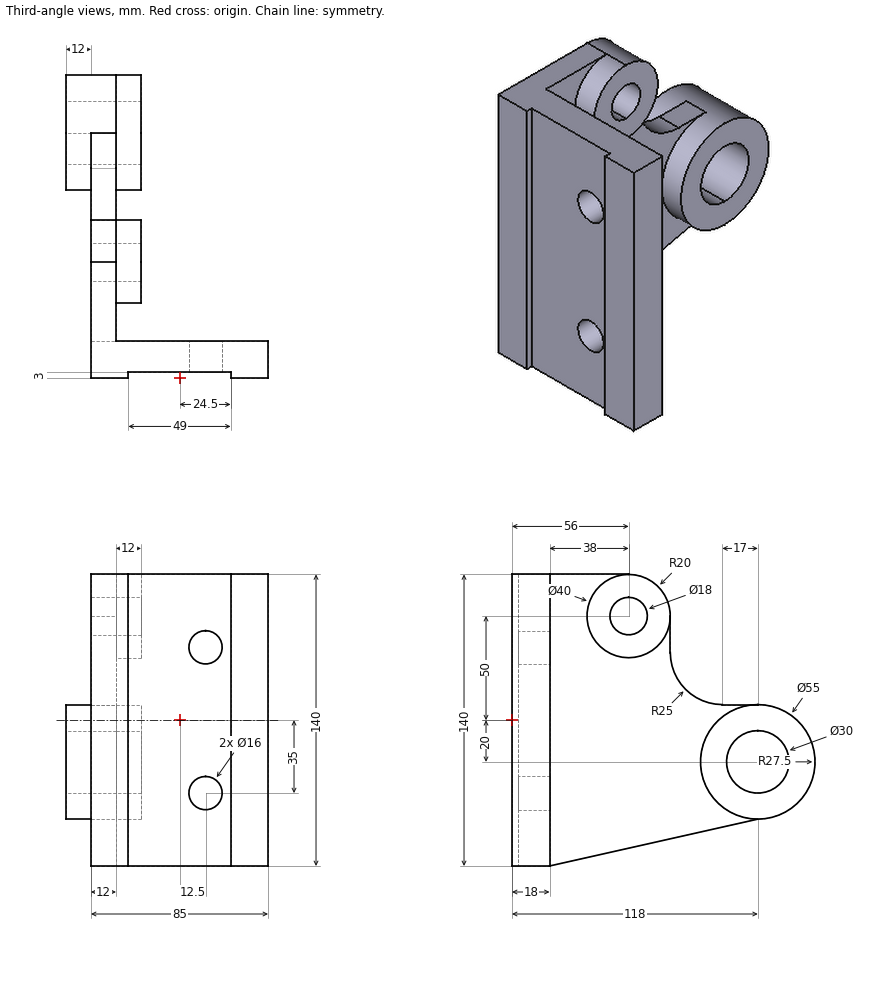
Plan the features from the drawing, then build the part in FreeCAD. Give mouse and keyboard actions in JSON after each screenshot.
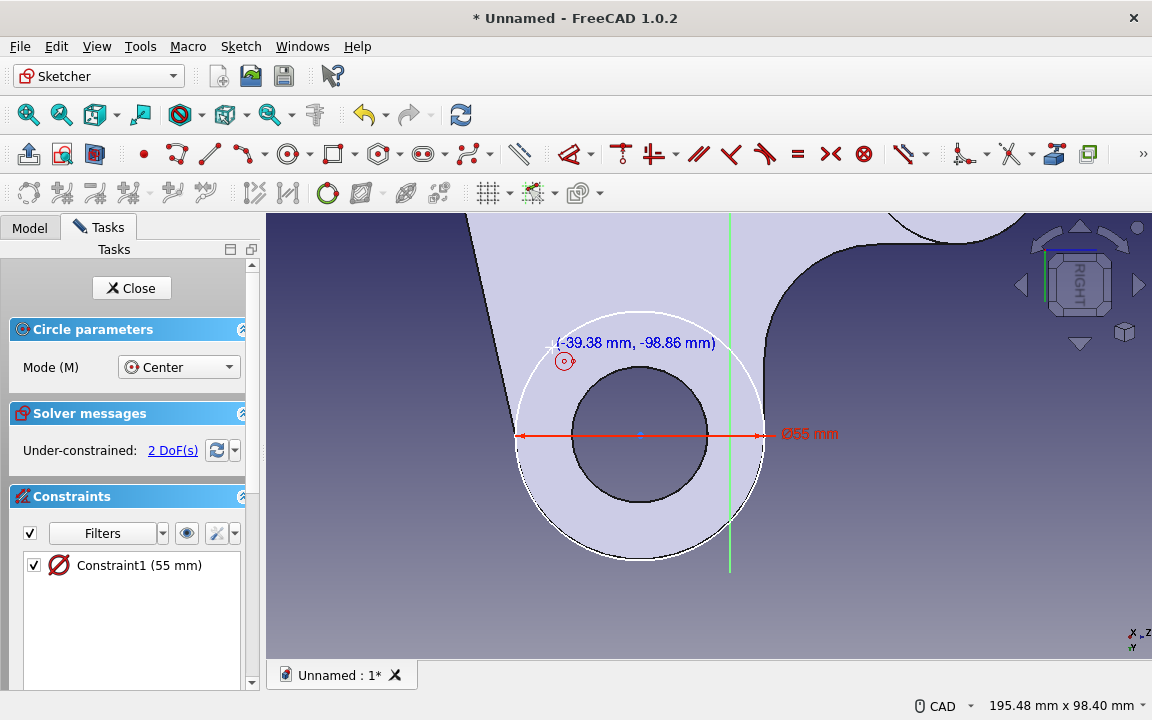
{"action": "left_click", "coordinate": [640, 436]}
{"action": "mouse_move", "coordinate": [688, 387]}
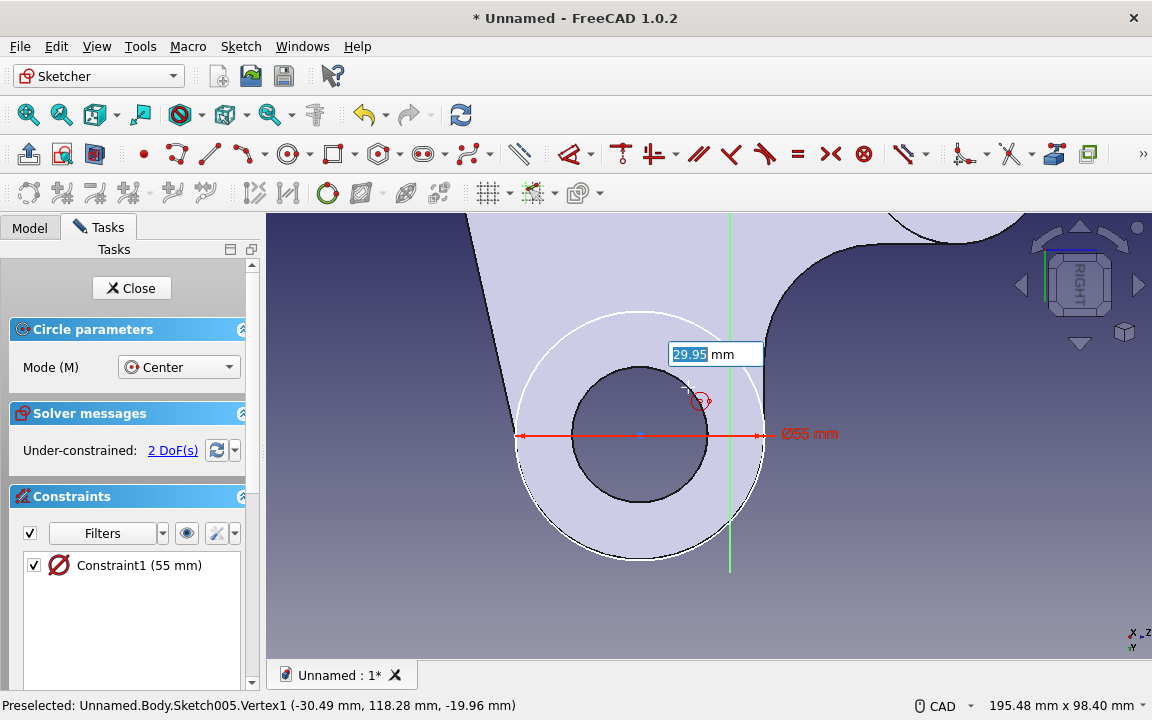
{"action": "type", "text": "30"}
{"action": "key", "text": "Return"}
{"action": "key", "text": "Escape"}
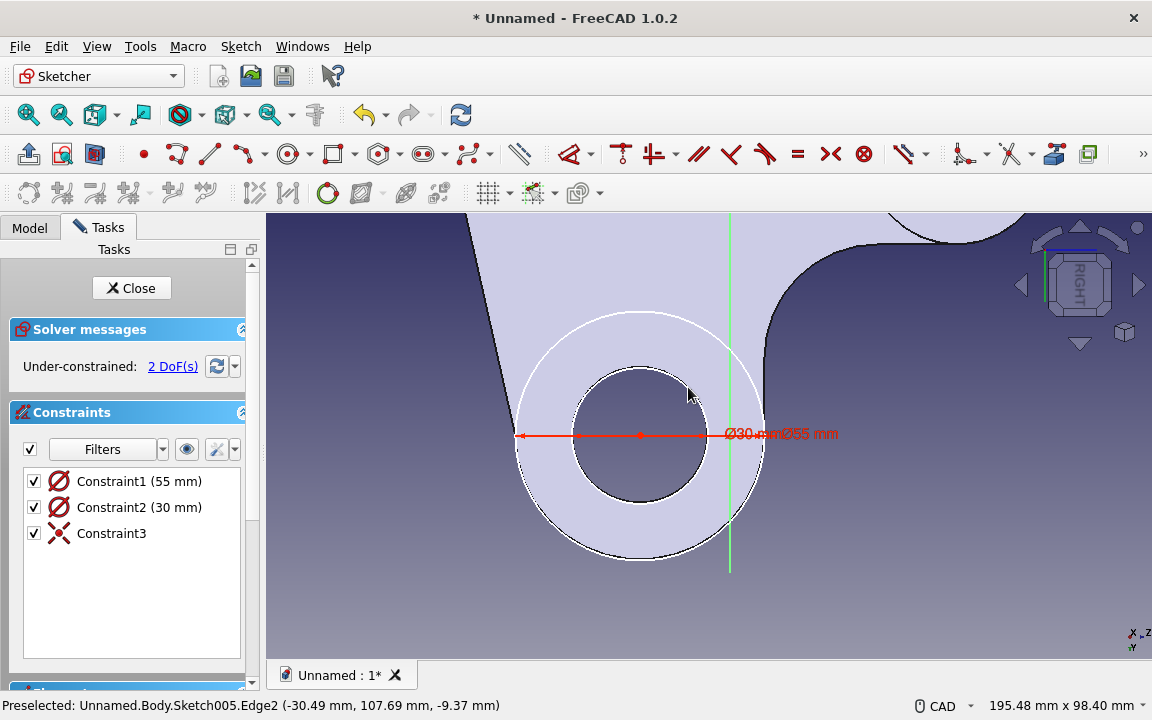
{"action": "left_click", "coordinate": [568, 154]}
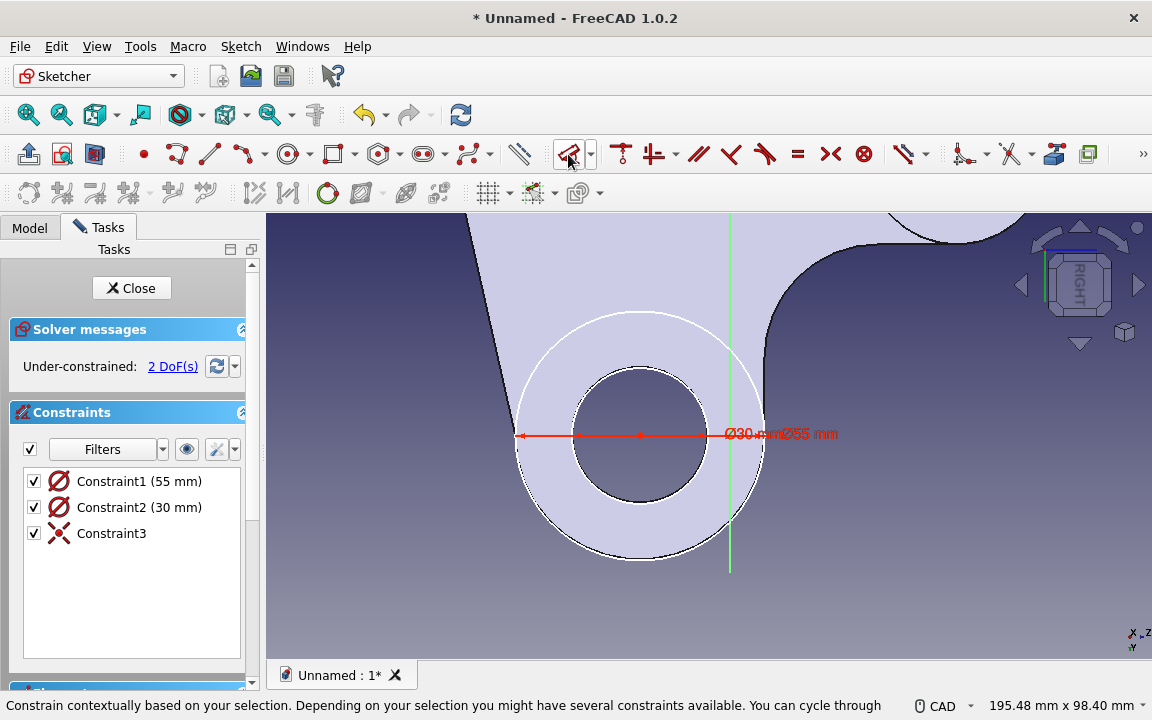
{"action": "left_click", "coordinate": [640, 436]}
{"action": "left_click", "coordinate": [664, 470]}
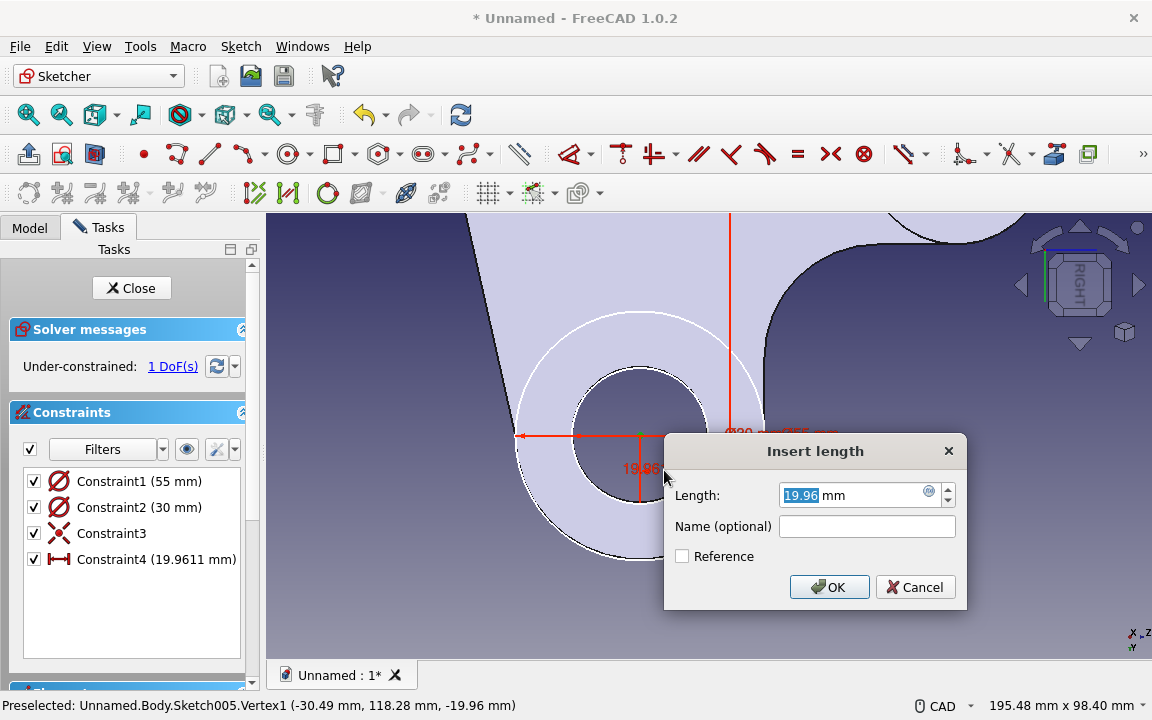
{"action": "type", "text": "20"}
{"action": "key", "text": "Return"}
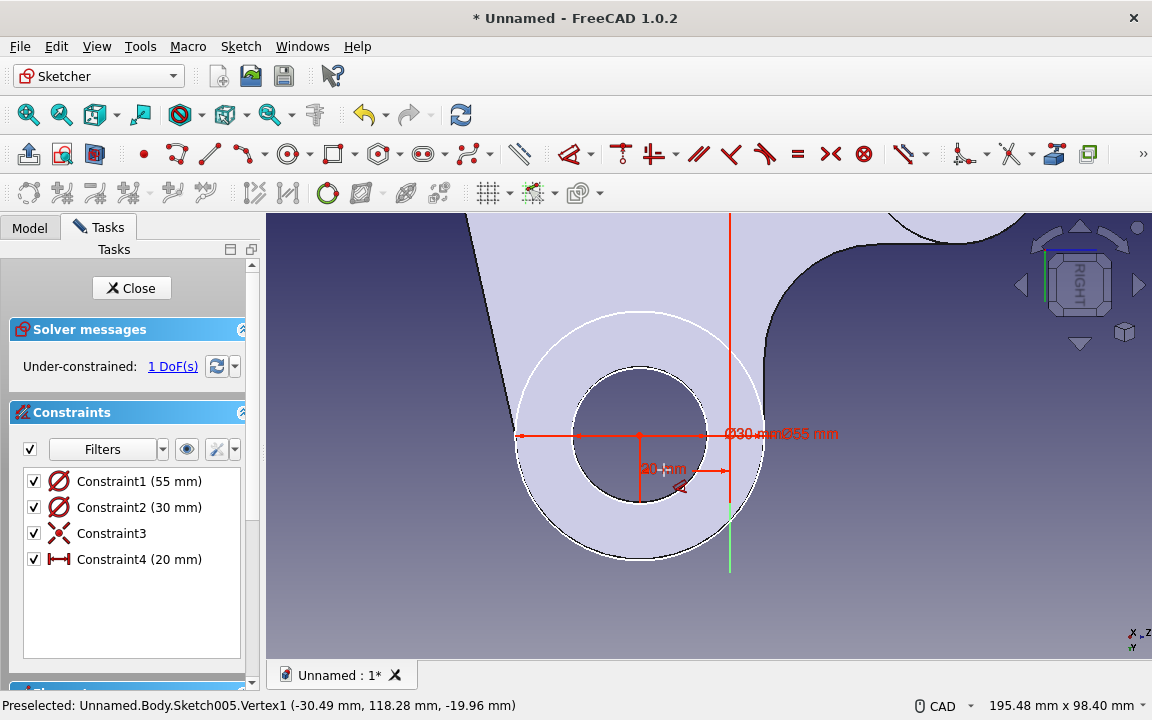
{"action": "left_click", "coordinate": [640, 436]}
{"action": "left_click", "coordinate": [764, 339]}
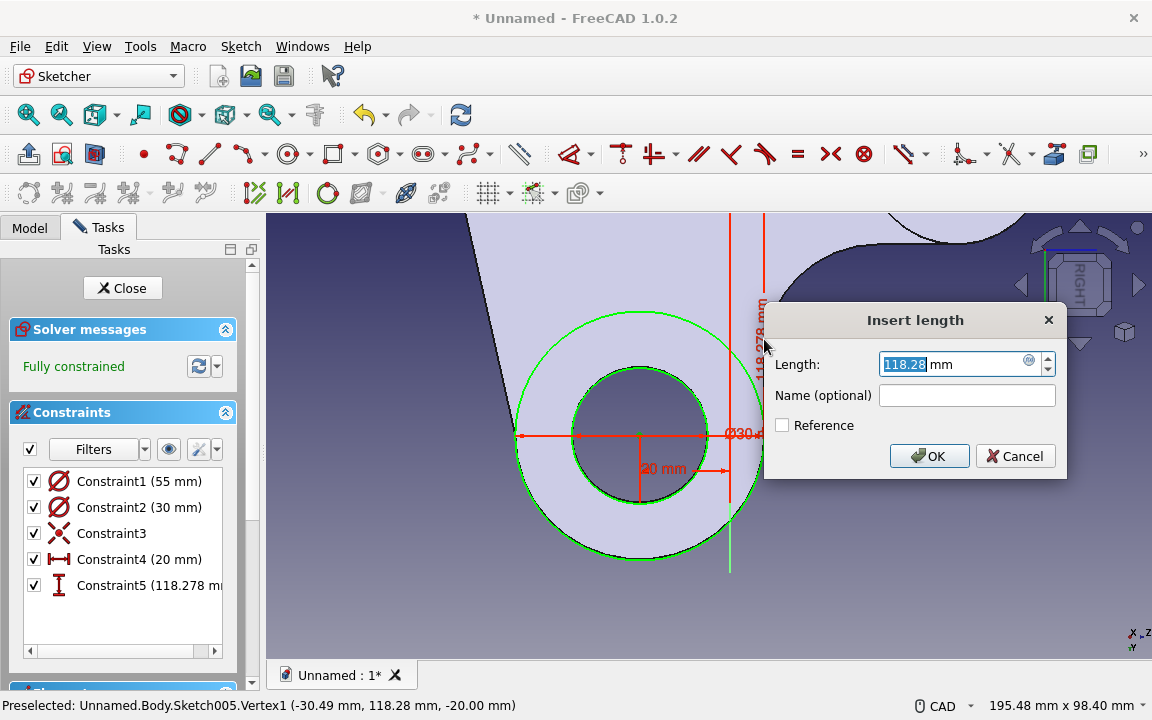
{"action": "type", "text": "118"}
{"action": "key", "text": "Return"}
{"action": "key", "text": "Escape"}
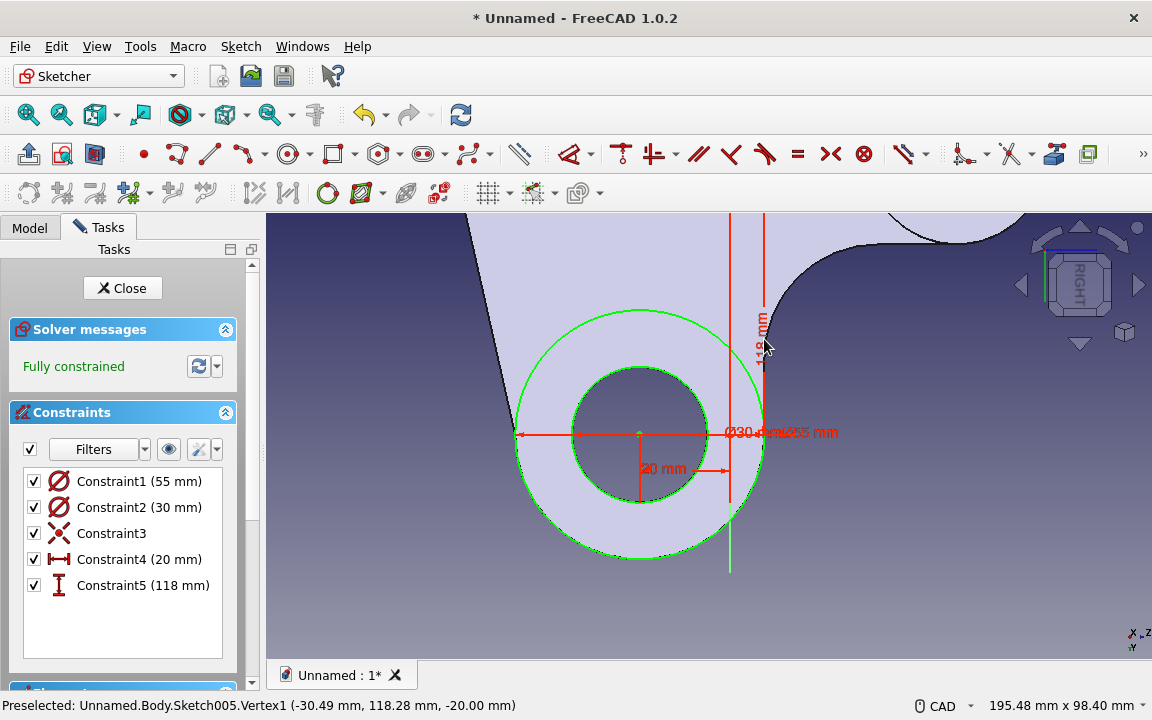
{"action": "left_click", "coordinate": [123, 288]}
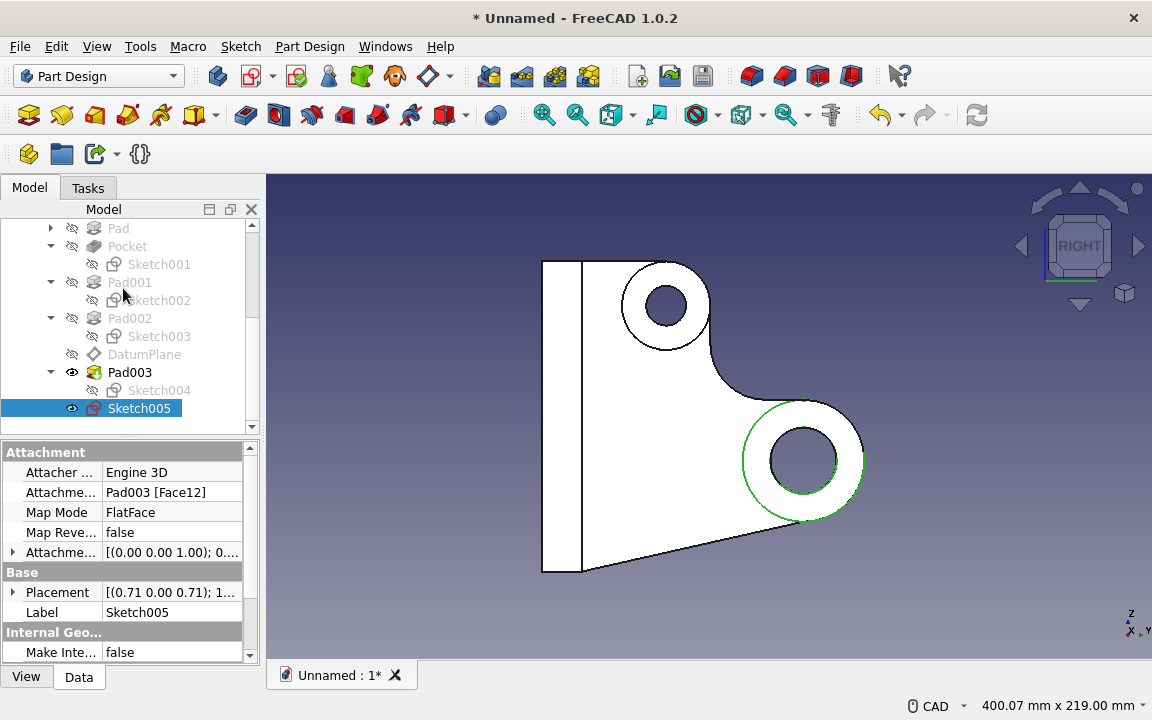
{"action": "left_click", "coordinate": [29, 116]}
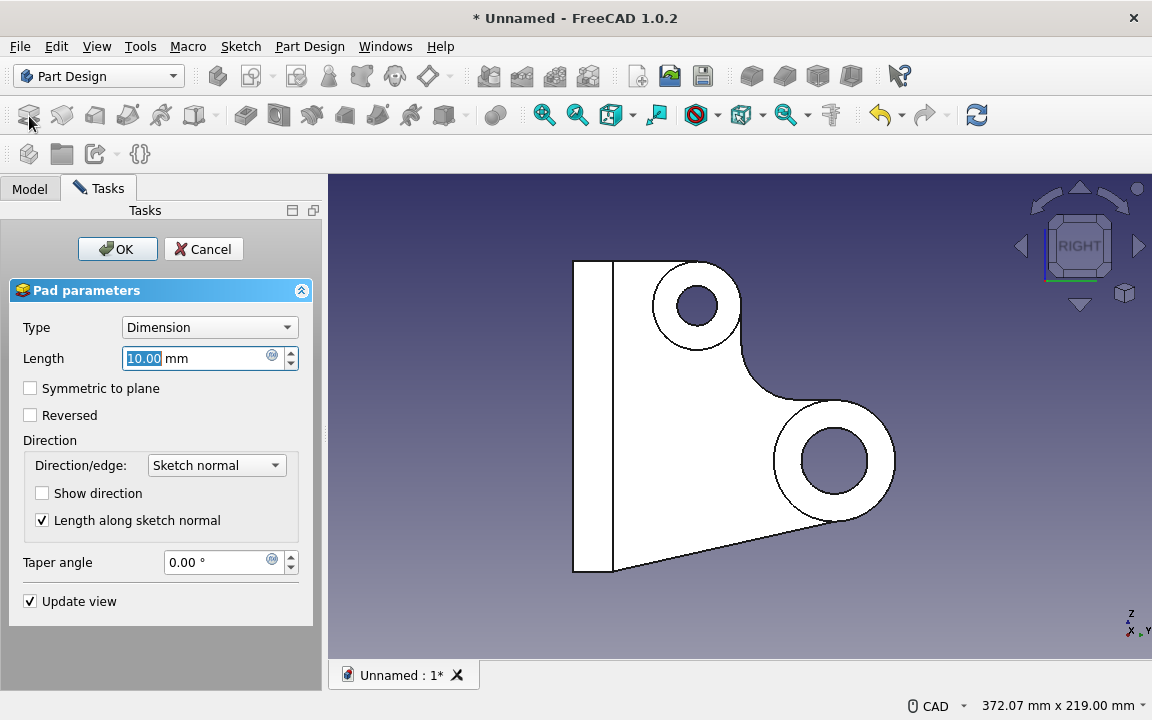
{"action": "type", "text": "12"}
{"action": "key", "text": "Tab"}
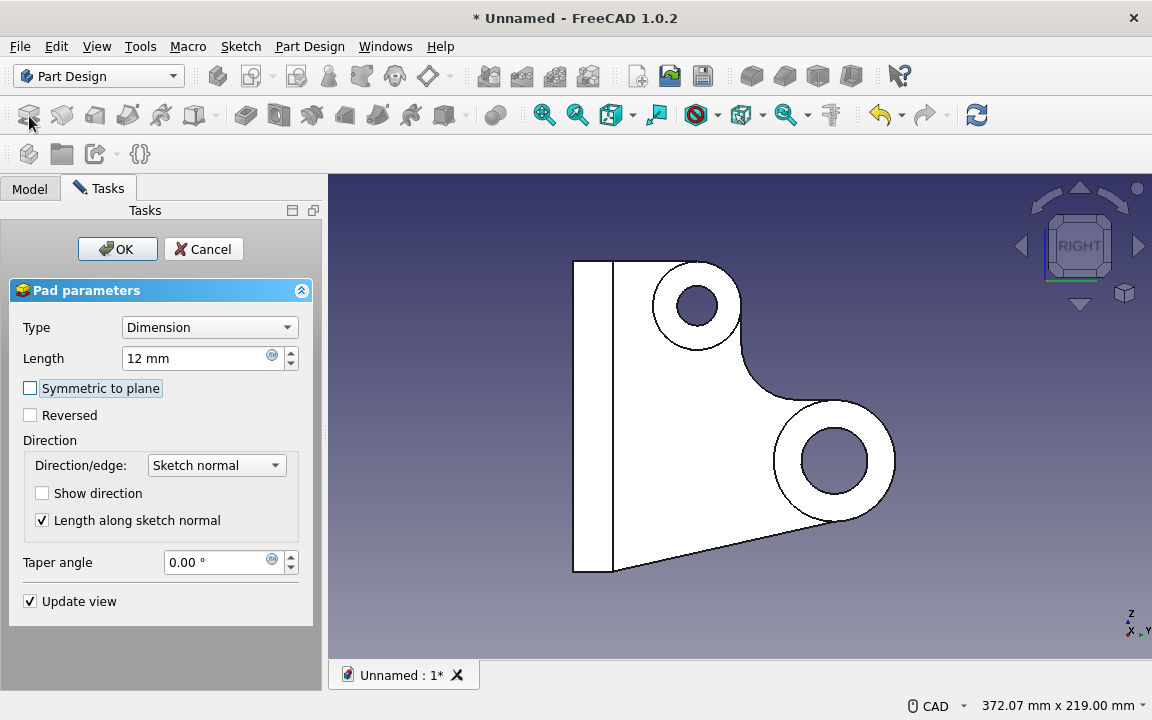
{"action": "left_click", "coordinate": [118, 249]}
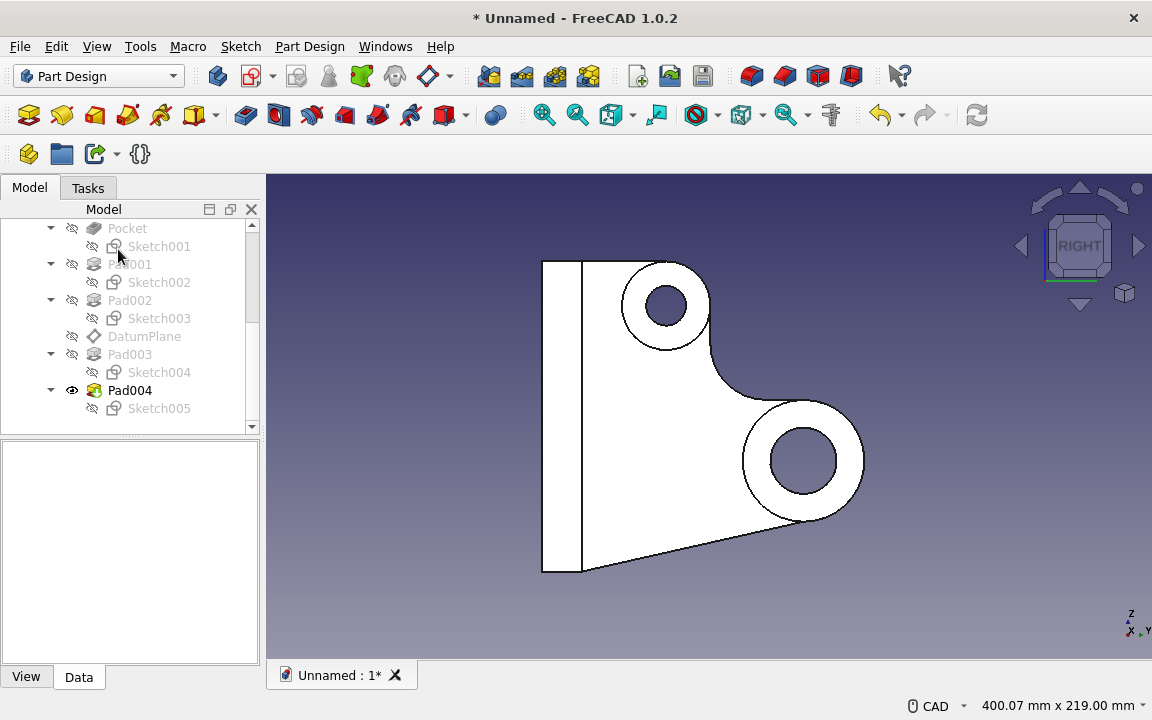
{"action": "key", "text": "4"}